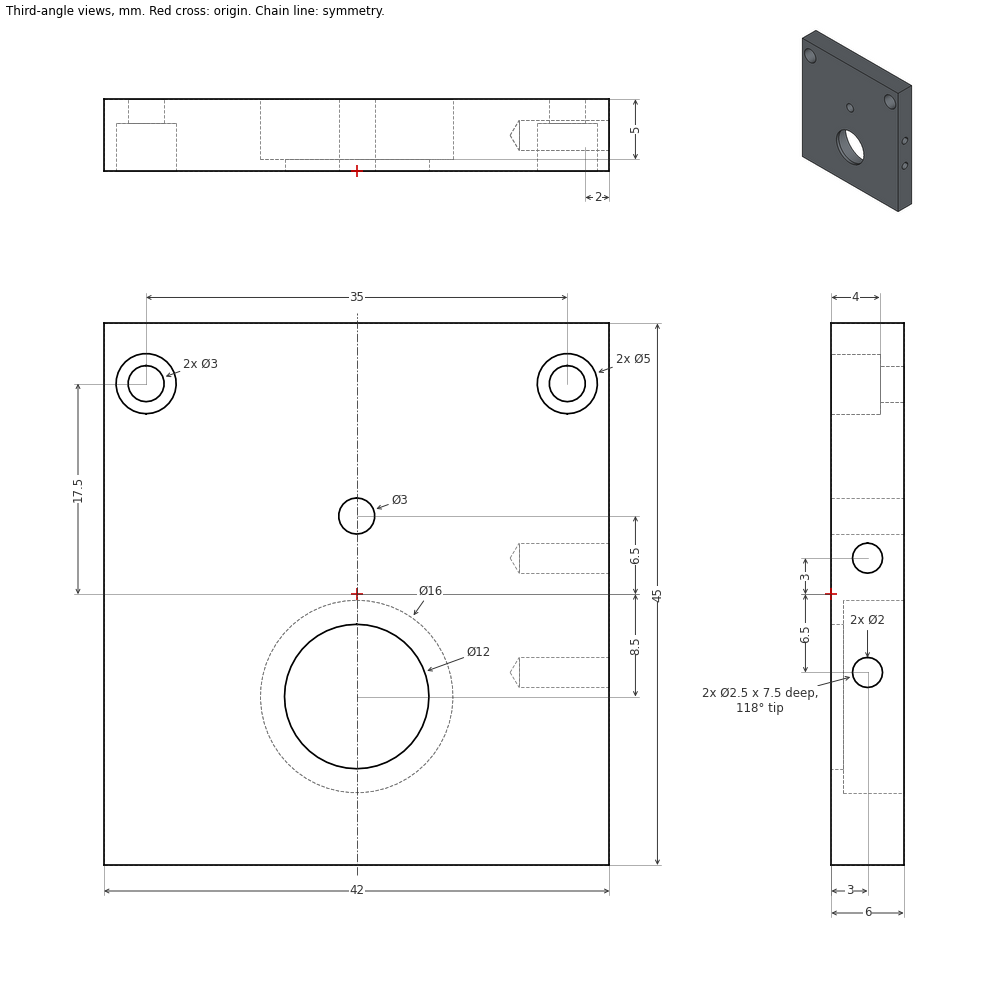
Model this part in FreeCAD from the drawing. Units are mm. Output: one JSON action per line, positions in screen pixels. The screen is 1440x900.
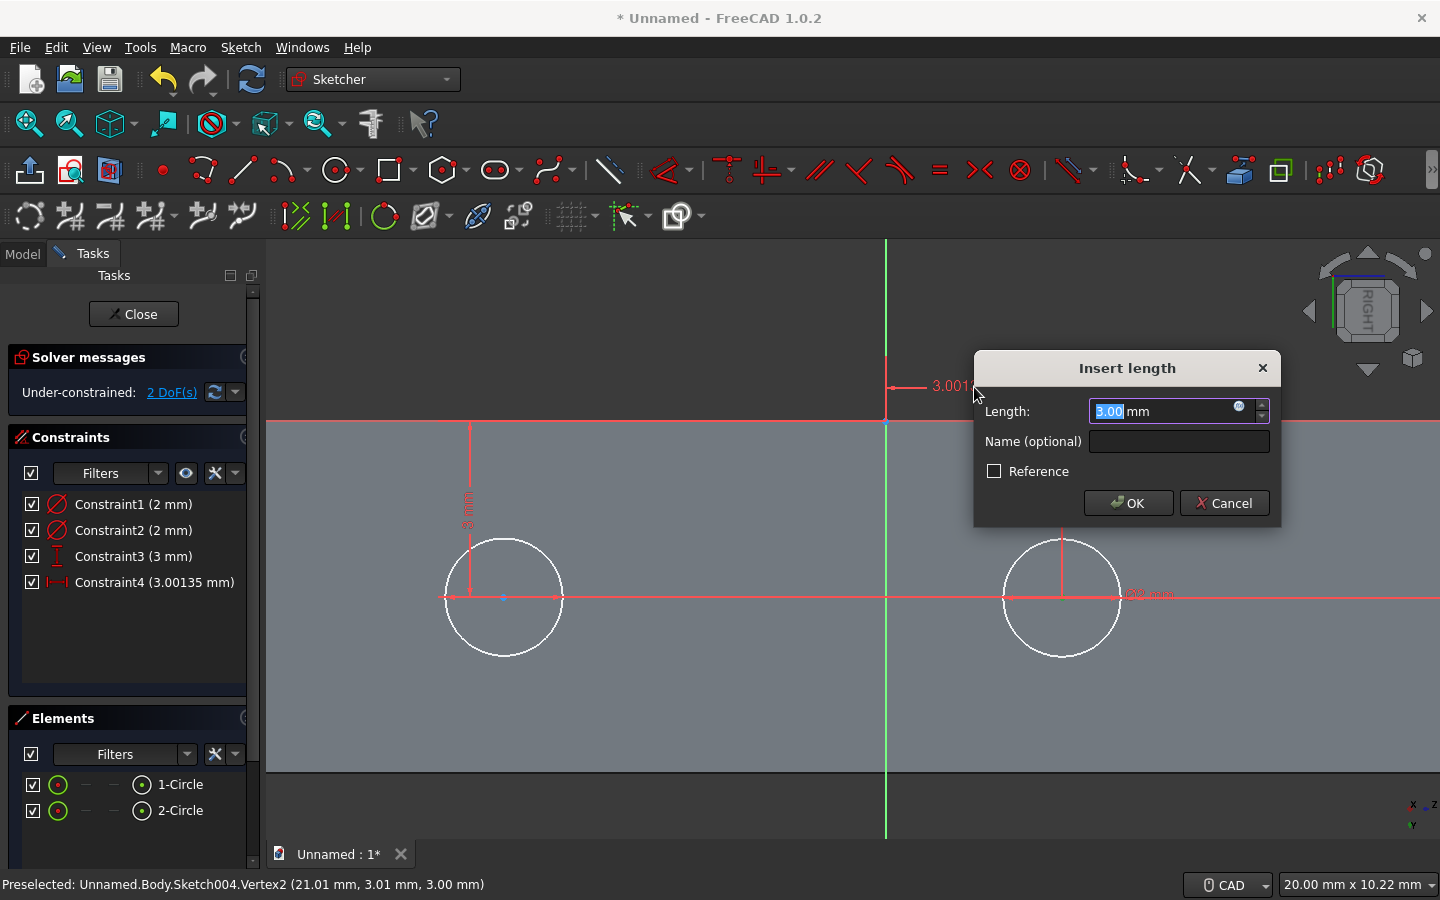
{"action": "type", "text": "3"}
{"action": "key", "text": "Return"}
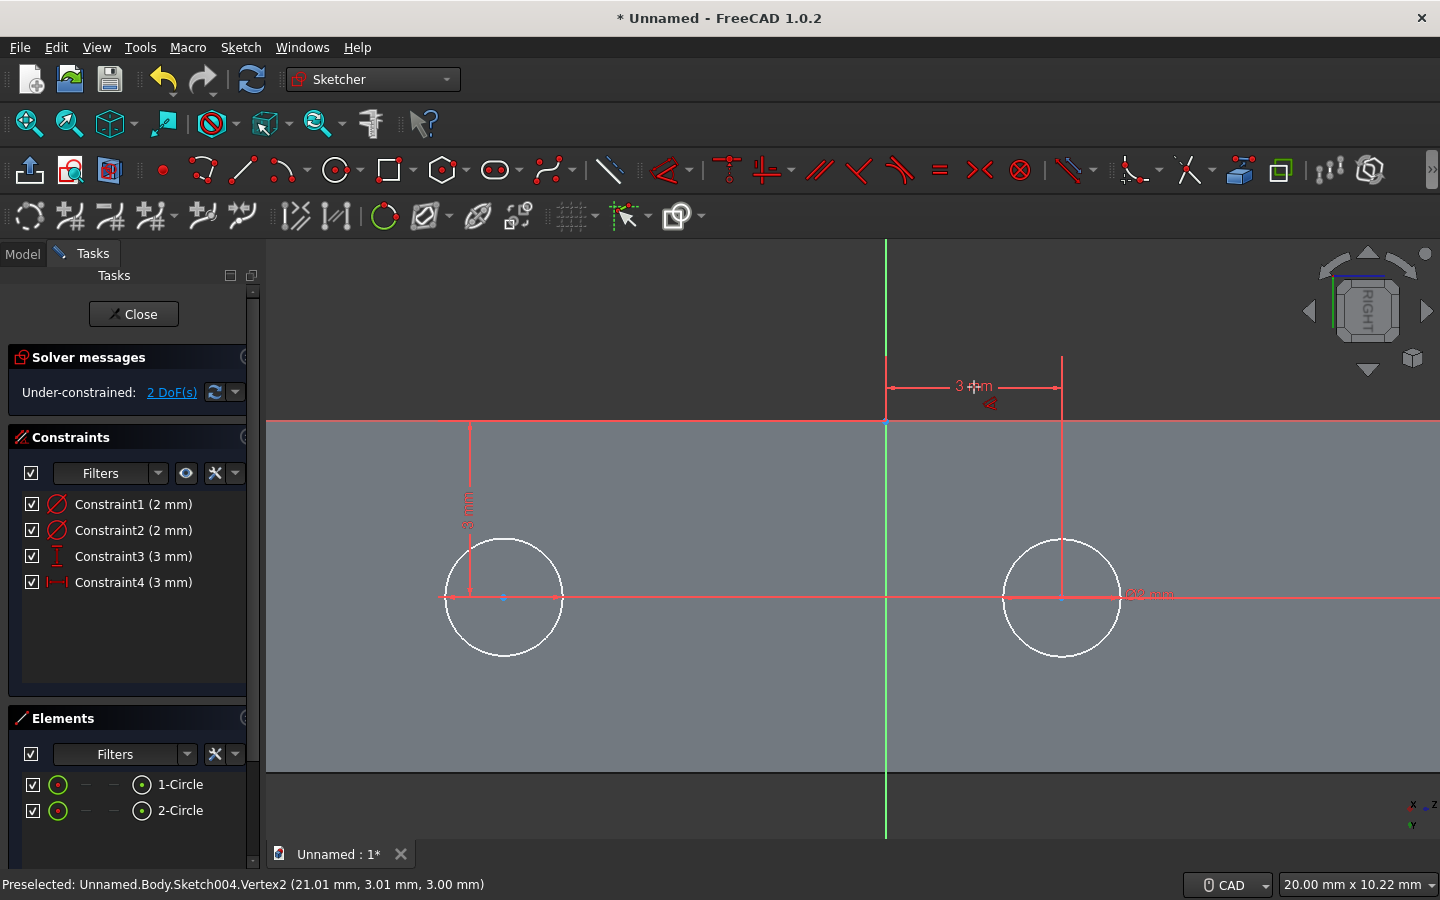
{"action": "left_click", "coordinate": [1062, 598]}
{"action": "left_click", "coordinate": [1096, 510]}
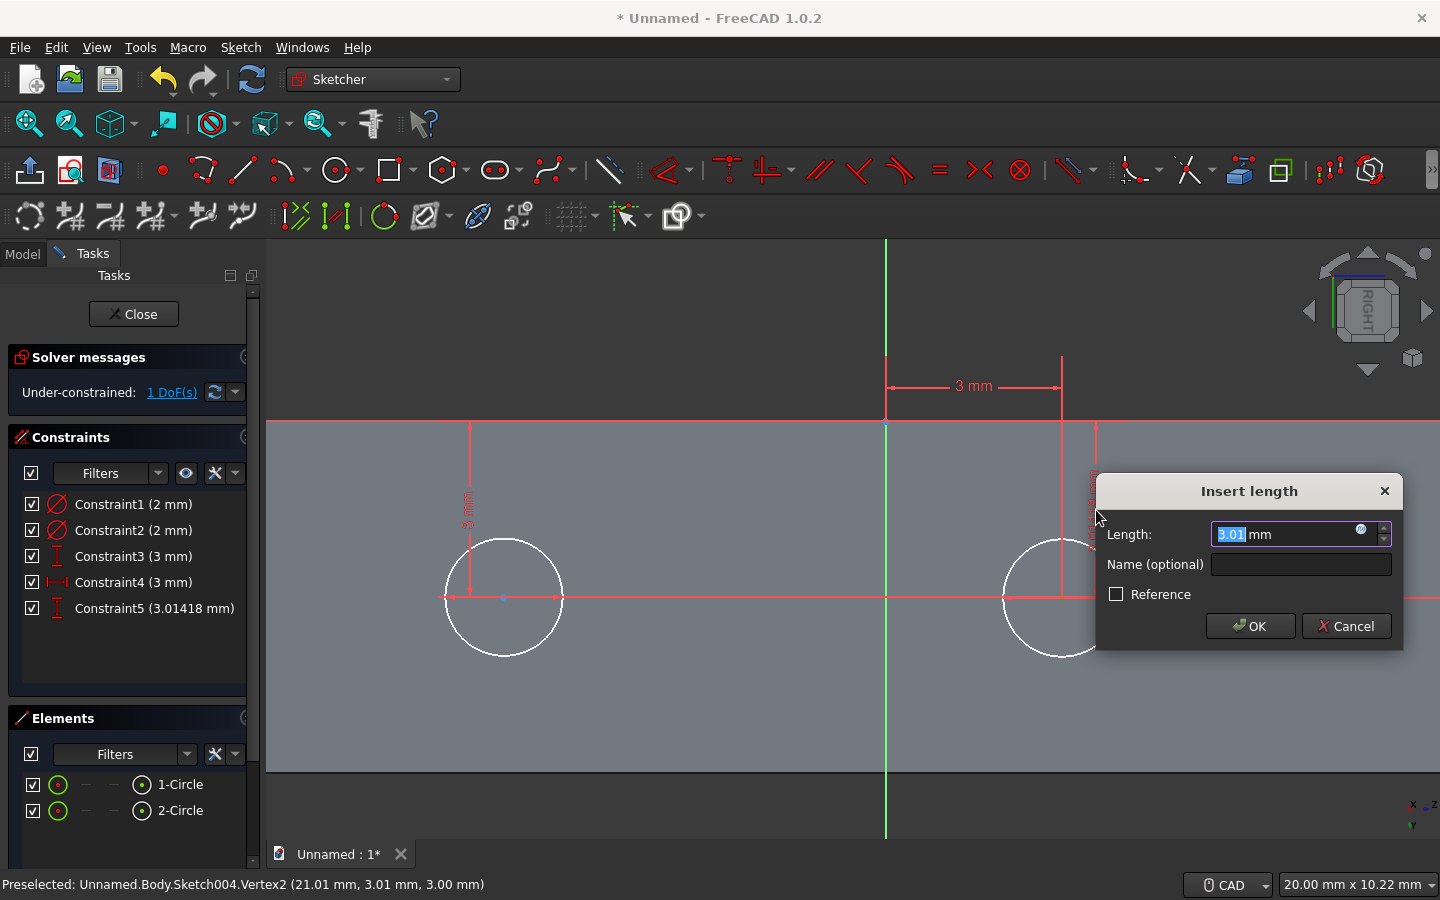
{"action": "type", "text": "3"}
{"action": "key", "text": "Return"}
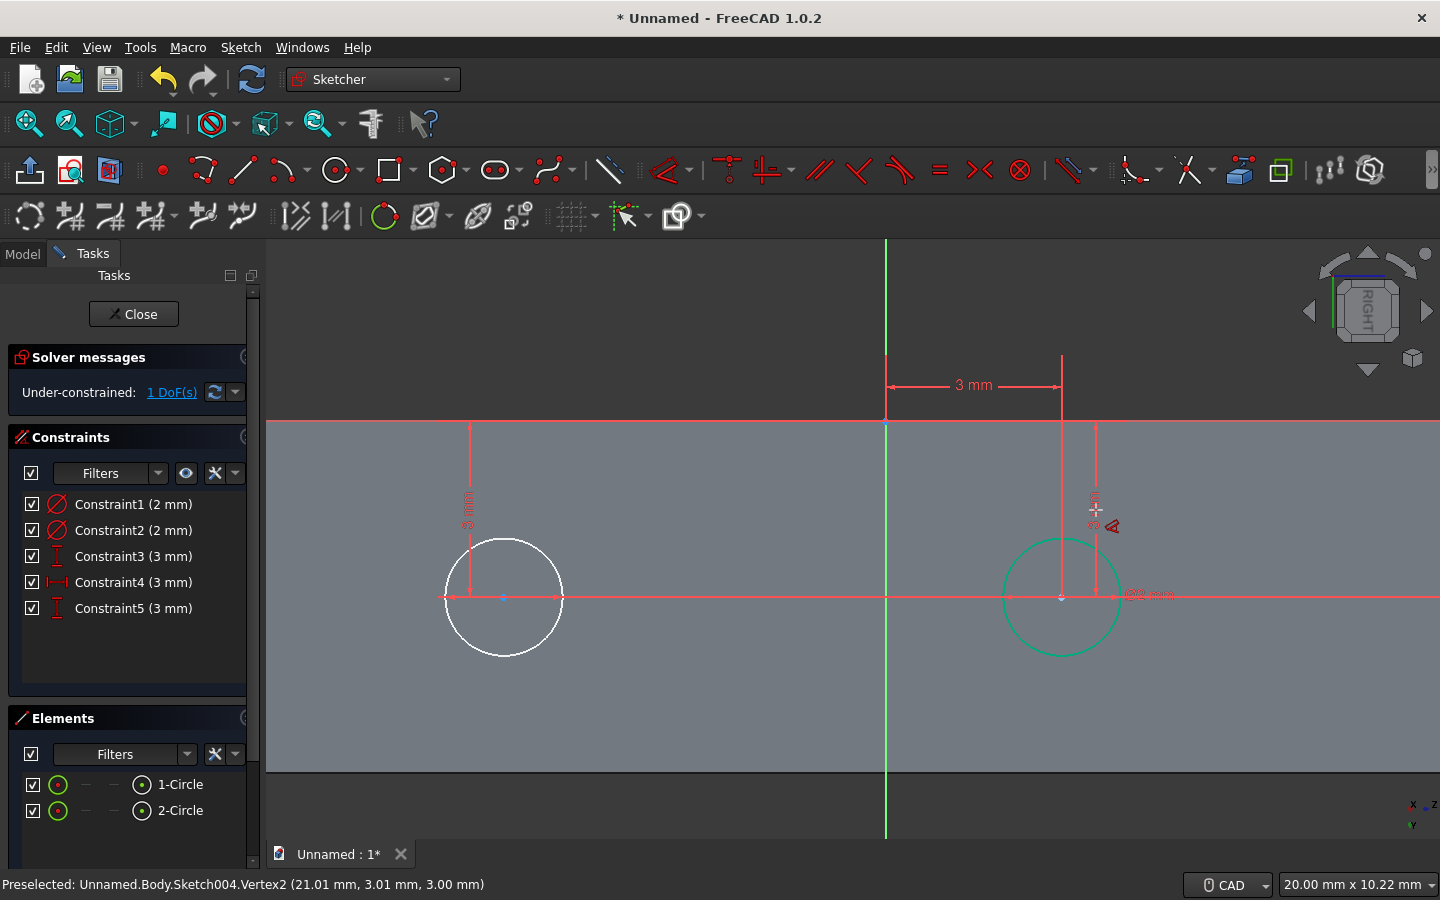
{"action": "left_click", "coordinate": [504, 597]}
{"action": "left_click", "coordinate": [695, 387]}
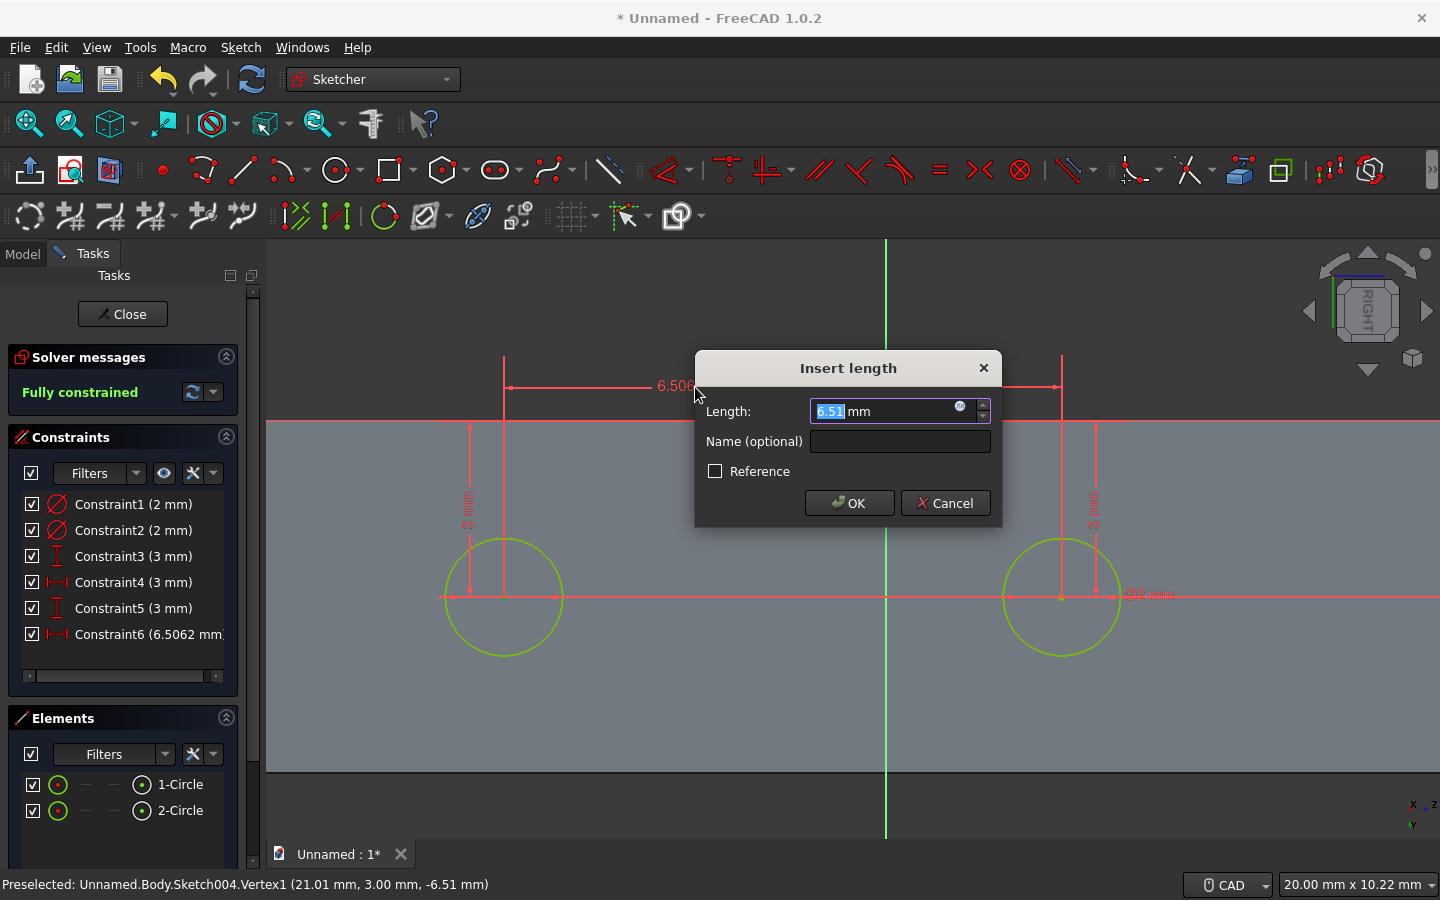
{"action": "type", "text": "6.5"}
{"action": "key", "text": "Return"}
{"action": "key", "text": "Escape"}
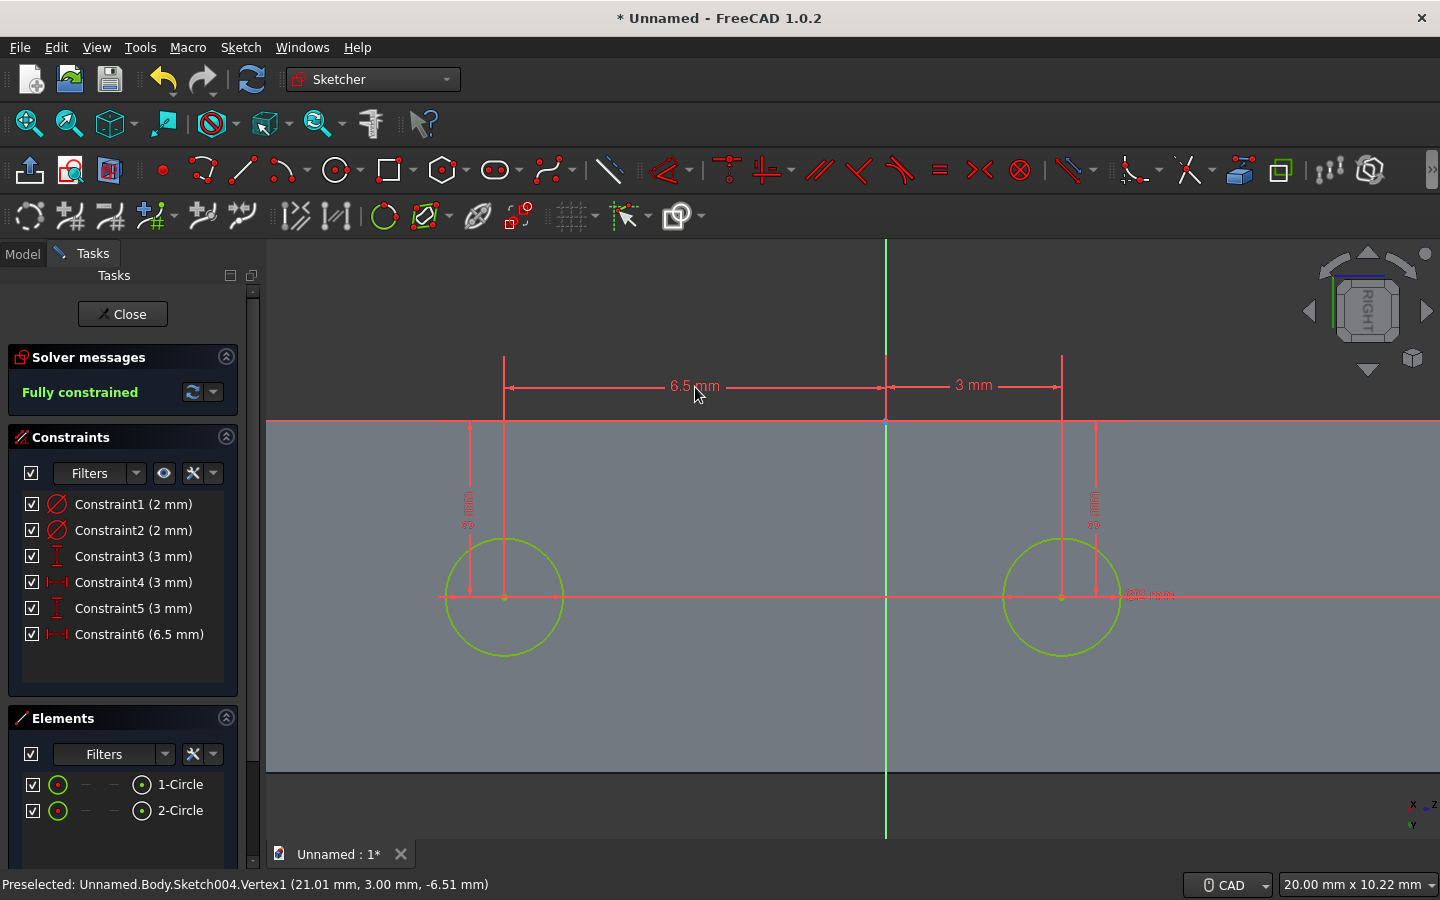
{"action": "left_click", "coordinate": [123, 314]}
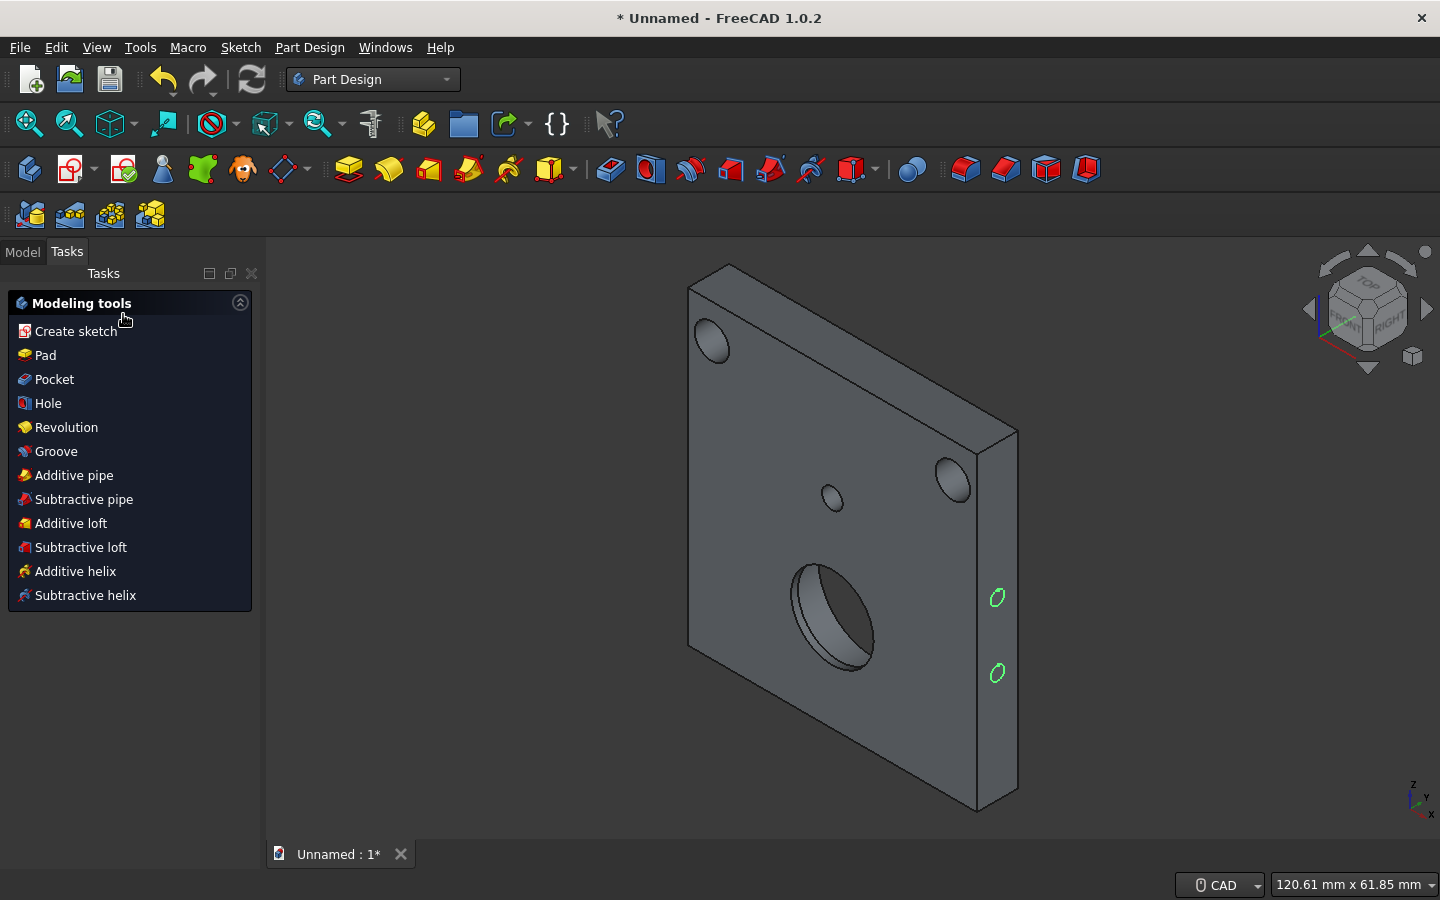
{"action": "left_click", "coordinate": [612, 170]}